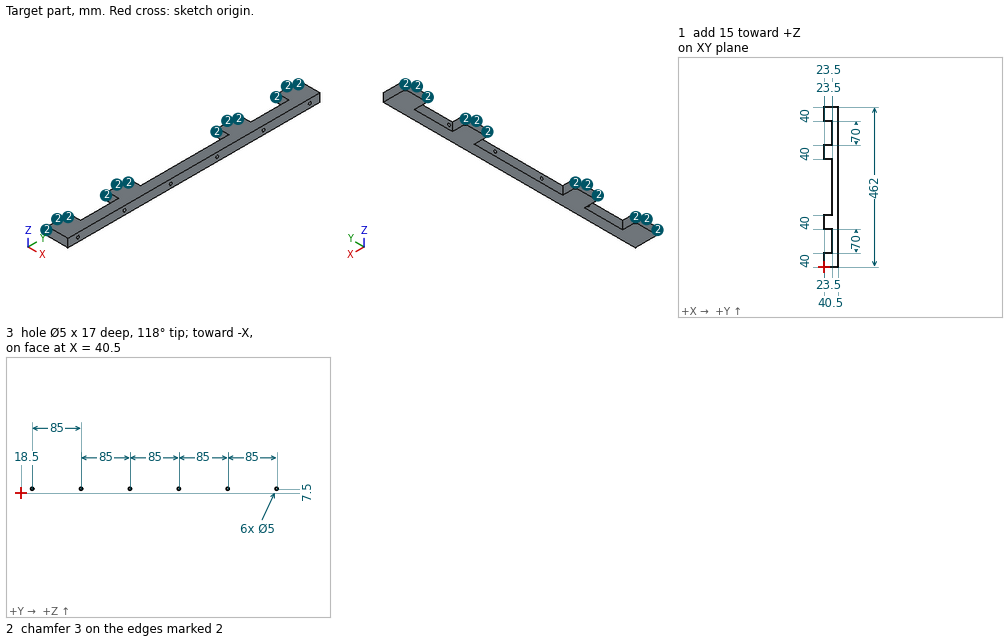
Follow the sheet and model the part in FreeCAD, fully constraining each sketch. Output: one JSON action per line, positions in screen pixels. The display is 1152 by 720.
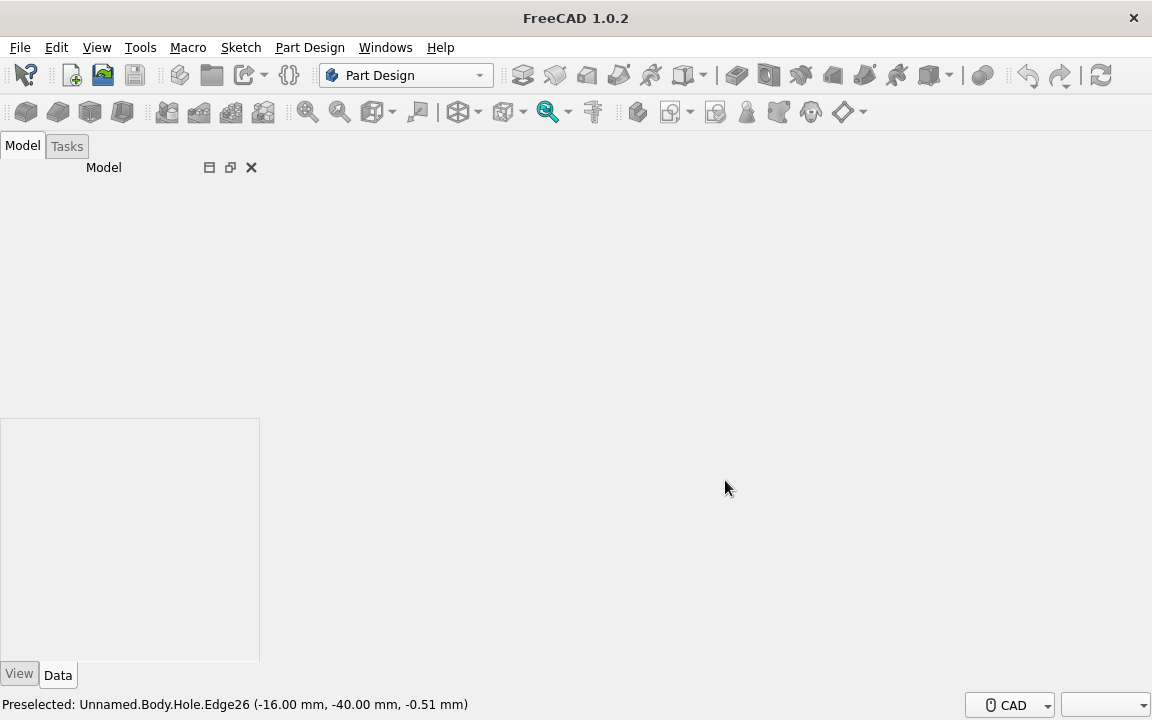
{"action": "left_click", "coordinate": [72, 76]}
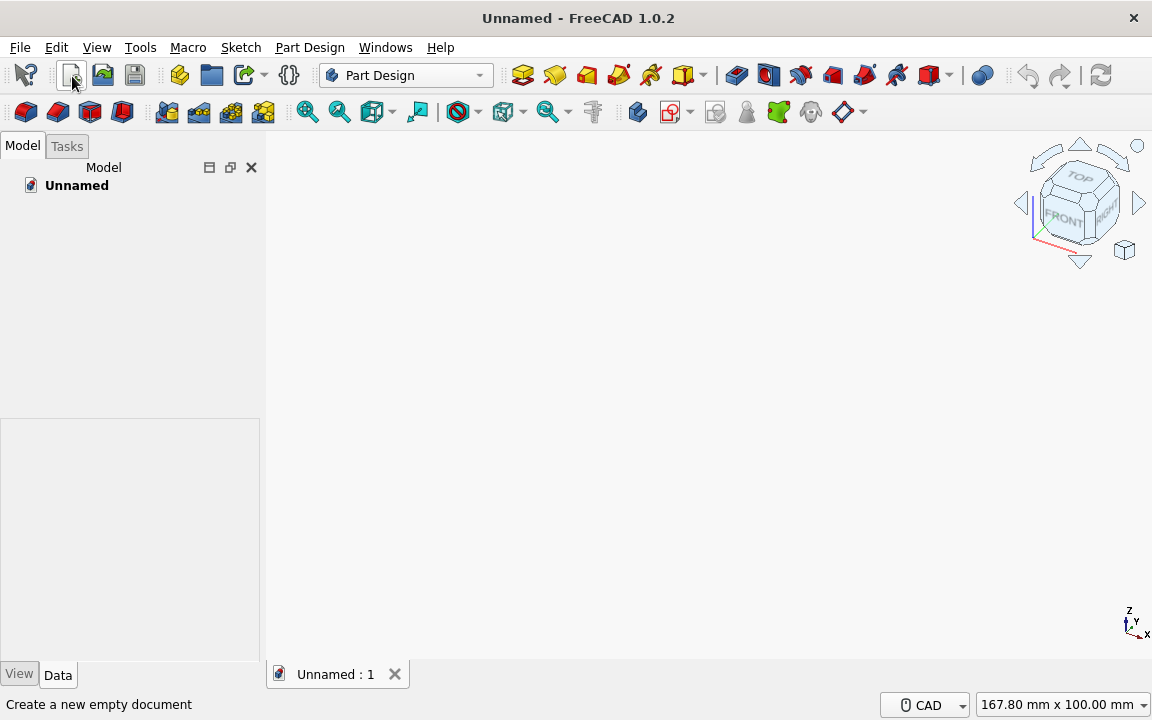
{"action": "left_click", "coordinate": [670, 112]}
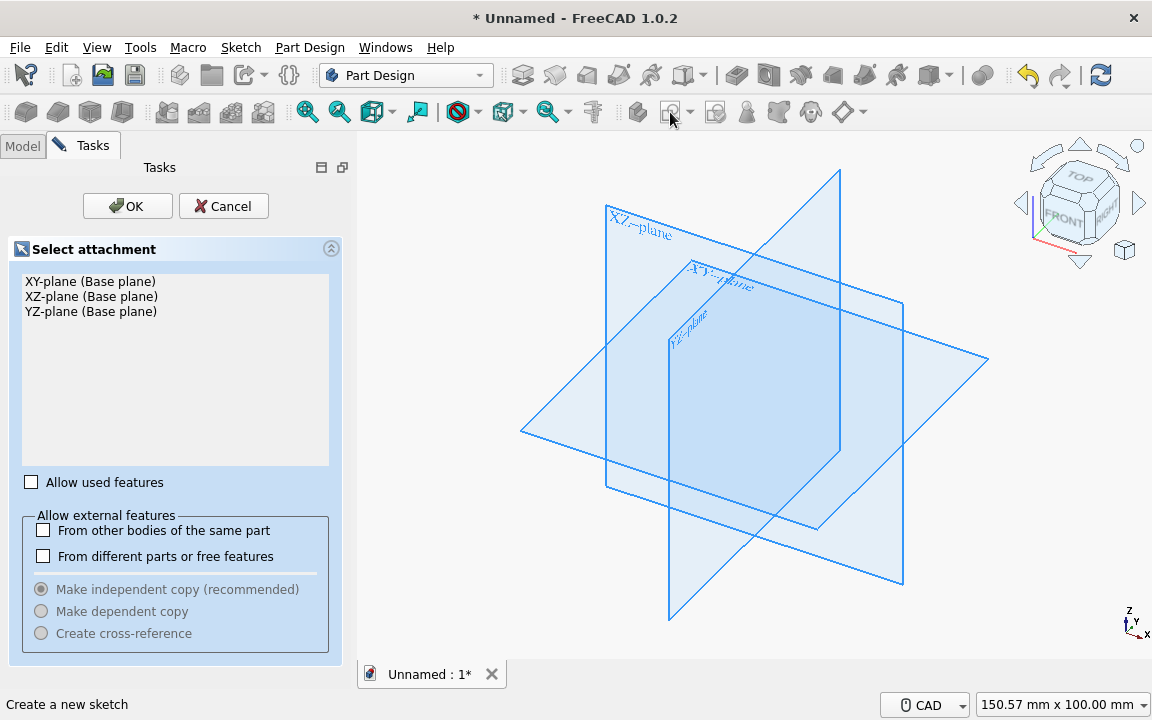
{"action": "left_click", "coordinate": [82, 282]}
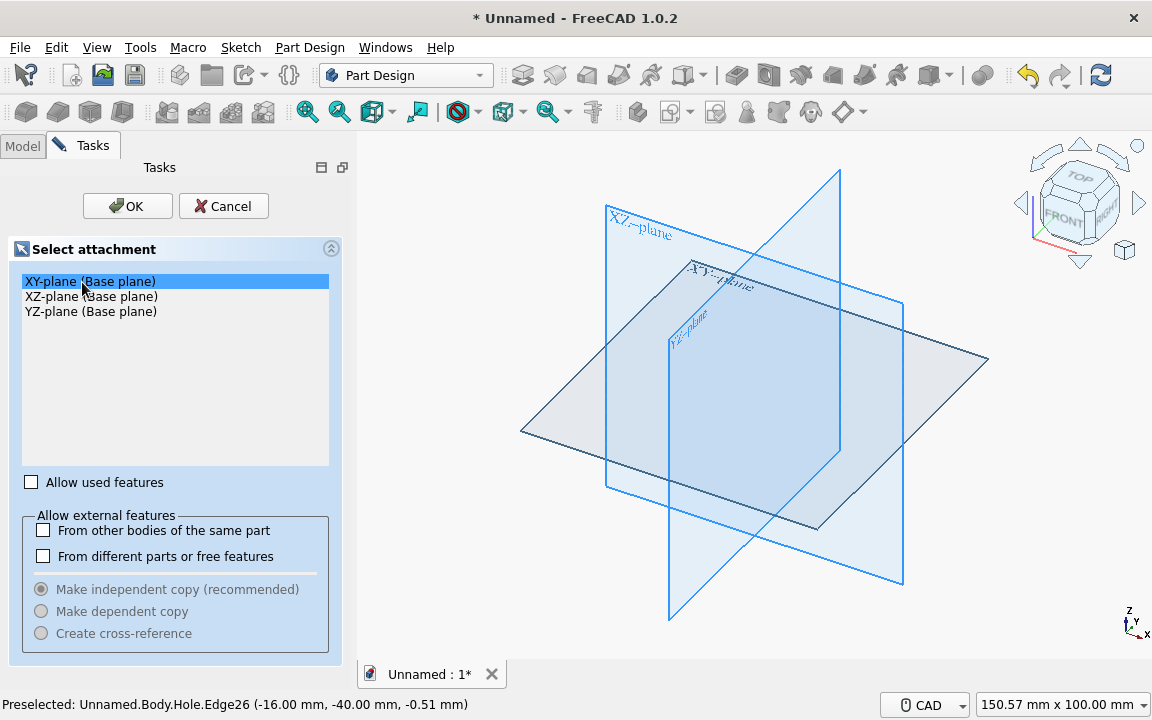
{"action": "left_click", "coordinate": [128, 206]}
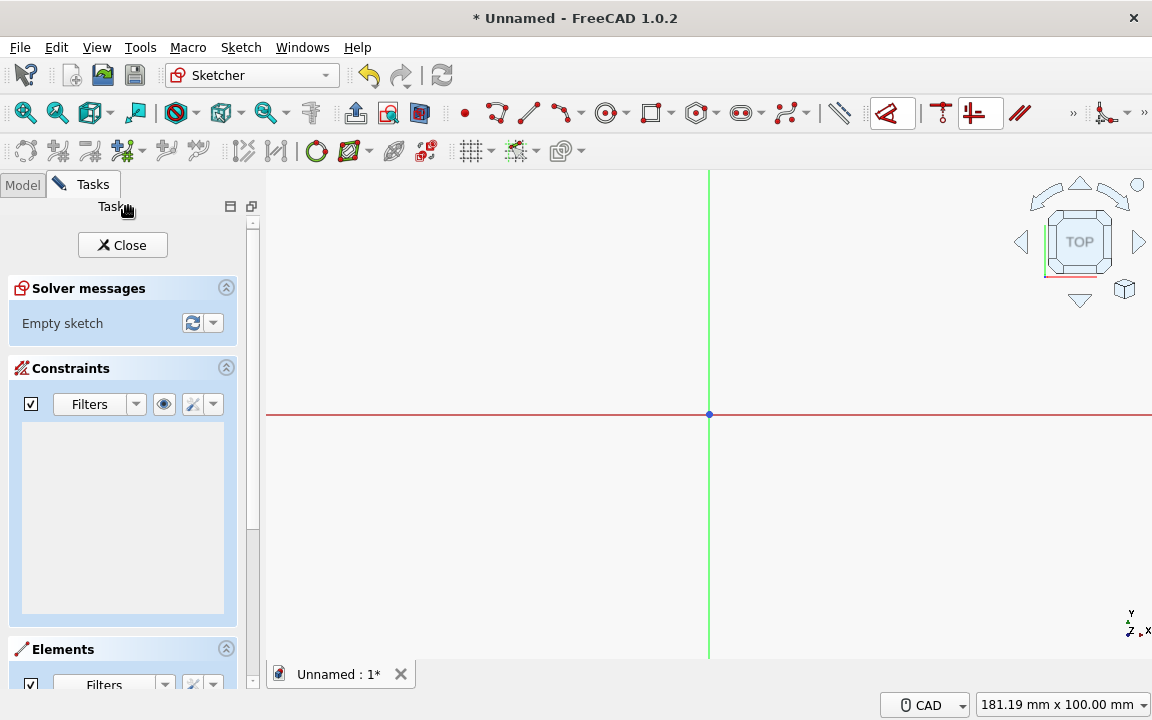
{"action": "scroll", "coordinate": [614, 591], "scroll_direction": "down", "scroll_amount": 10}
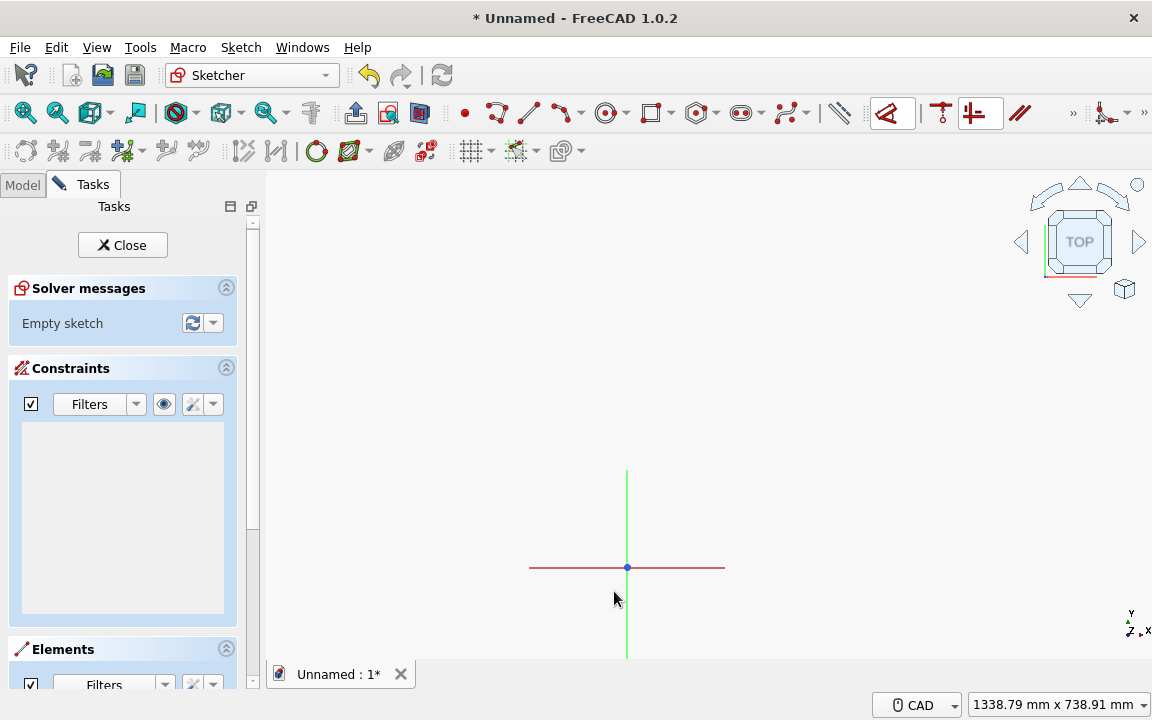
{"action": "left_click", "coordinate": [498, 114]}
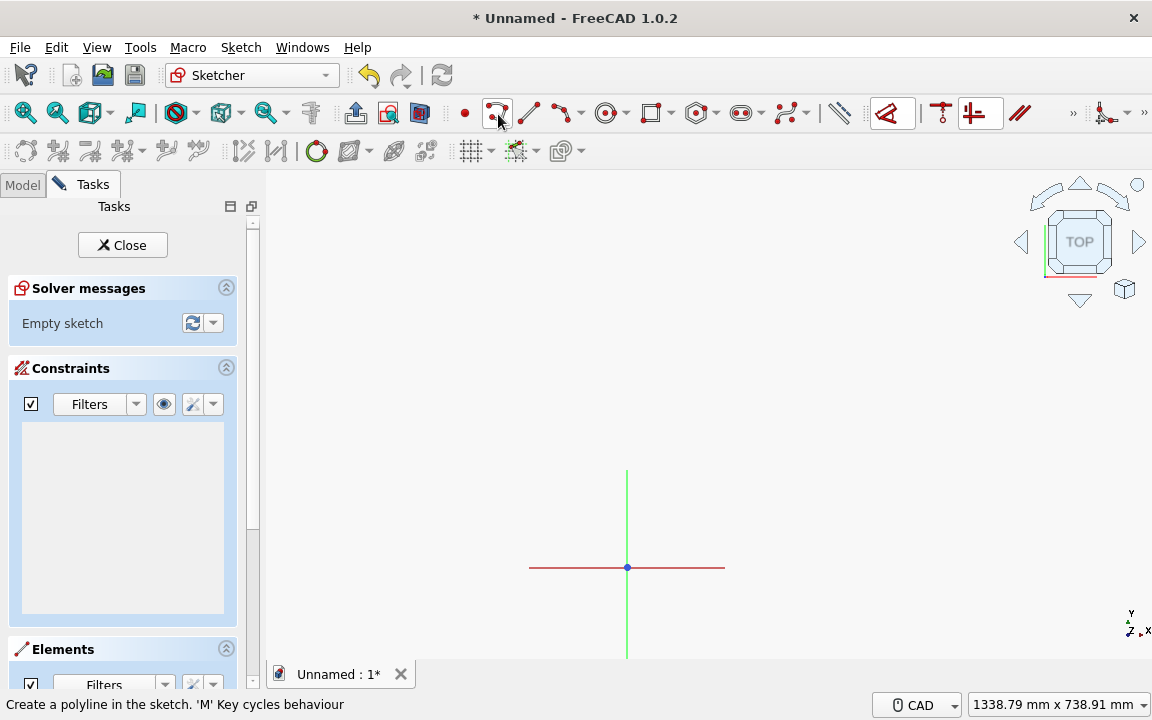
{"action": "left_click", "coordinate": [627, 568]}
{"action": "left_click", "coordinate": [654, 559]}
{"action": "left_click", "coordinate": [654, 262]}
{"action": "left_click", "coordinate": [627, 262]}
{"action": "left_click", "coordinate": [636, 289]}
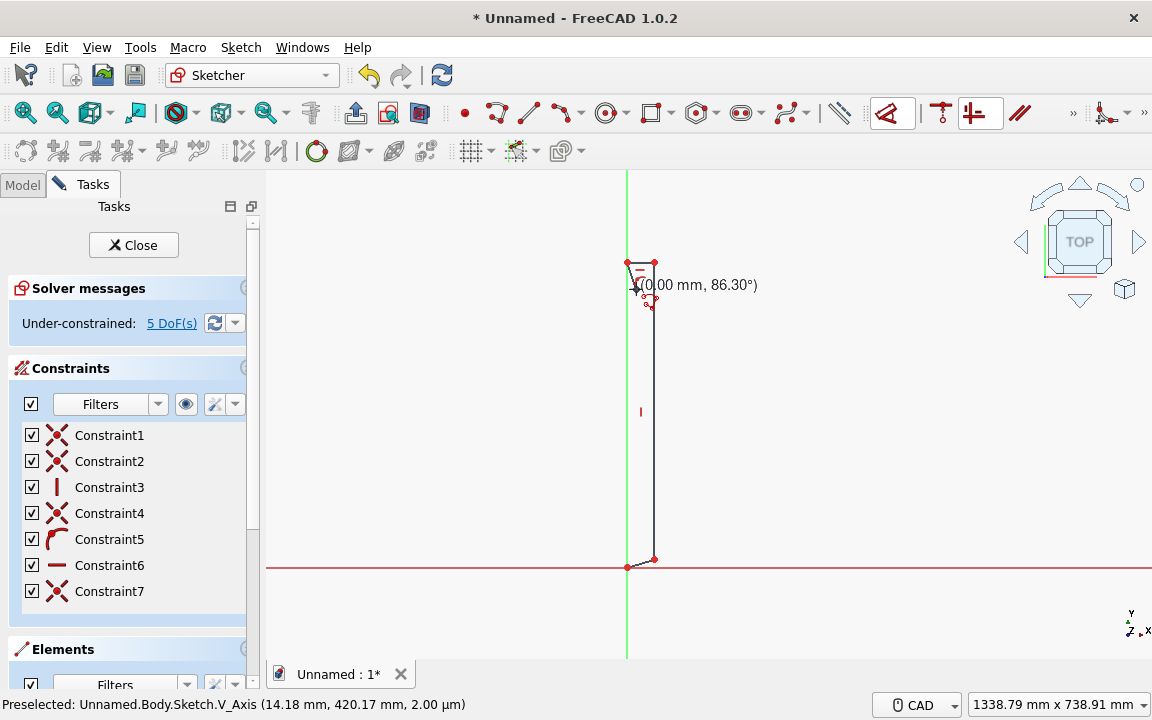
{"action": "scroll", "coordinate": [643, 289], "scroll_direction": "up", "scroll_amount": 2}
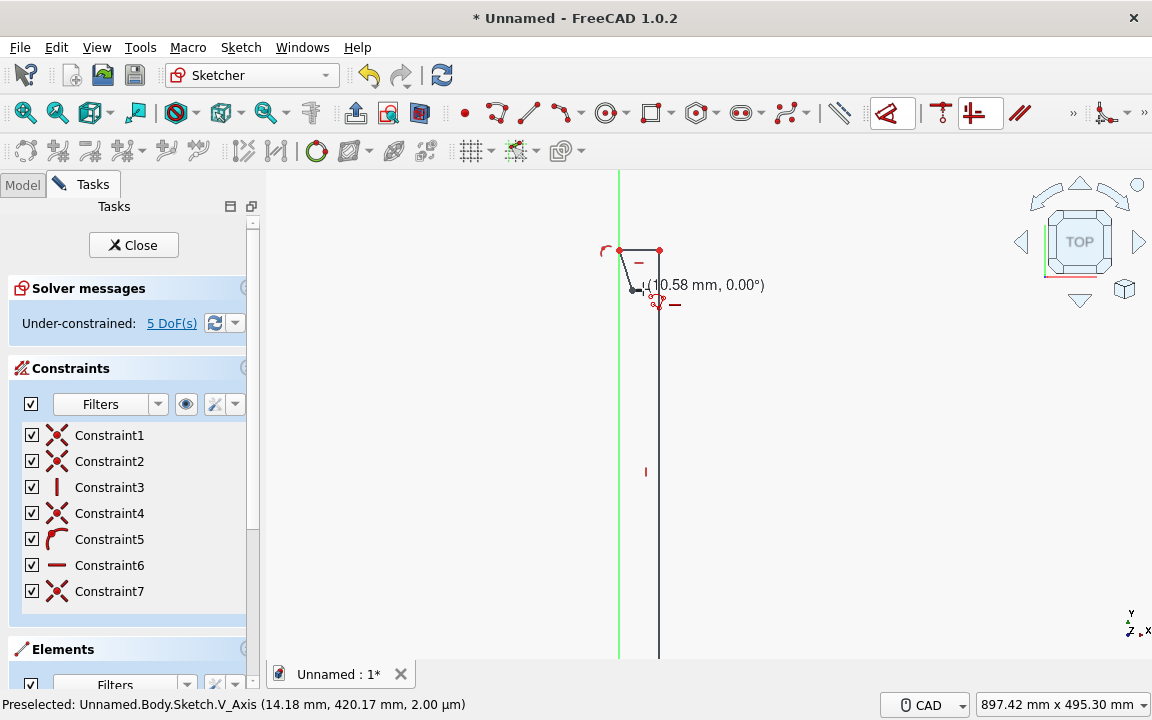
{"action": "left_click", "coordinate": [642, 289]}
{"action": "left_click", "coordinate": [642, 357]}
{"action": "left_click", "coordinate": [619, 357]}
{"action": "left_click", "coordinate": [628, 397]}
{"action": "left_click", "coordinate": [642, 397]}
{"action": "left_click", "coordinate": [642, 557]}
{"action": "left_click", "coordinate": [619, 557]}
{"action": "left_click", "coordinate": [628, 596]}
{"action": "left_click", "coordinate": [642, 596]}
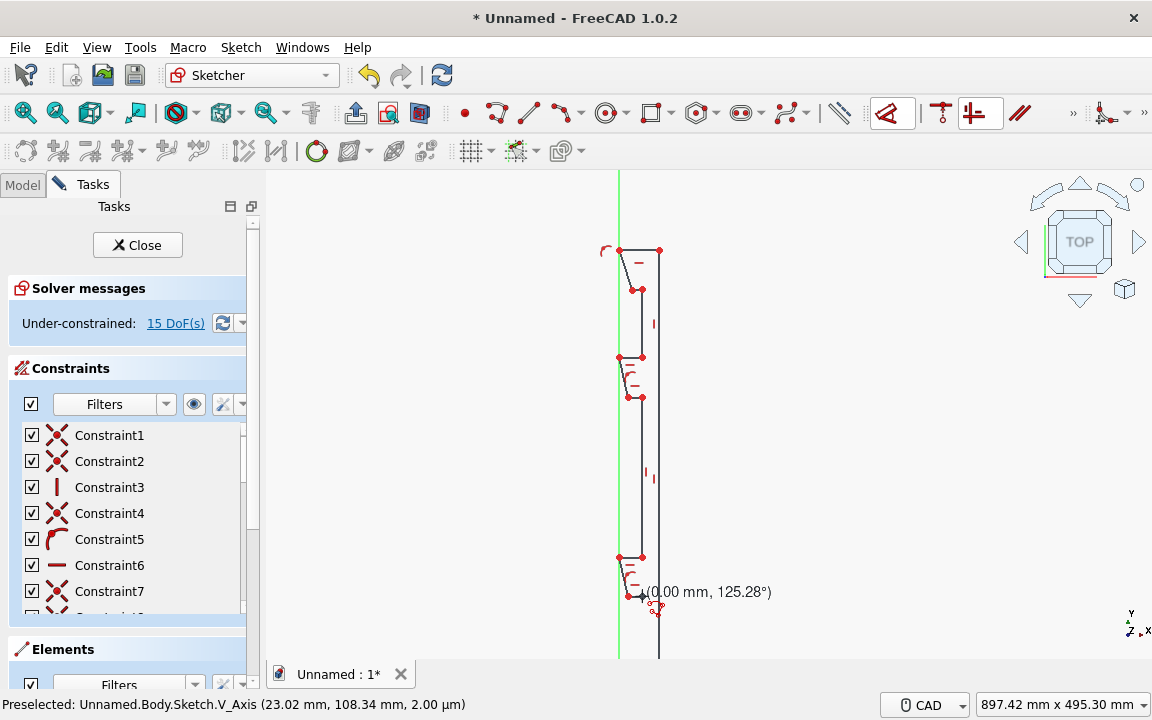
{"action": "scroll", "coordinate": [643, 288], "scroll_direction": "down", "scroll_amount": 2}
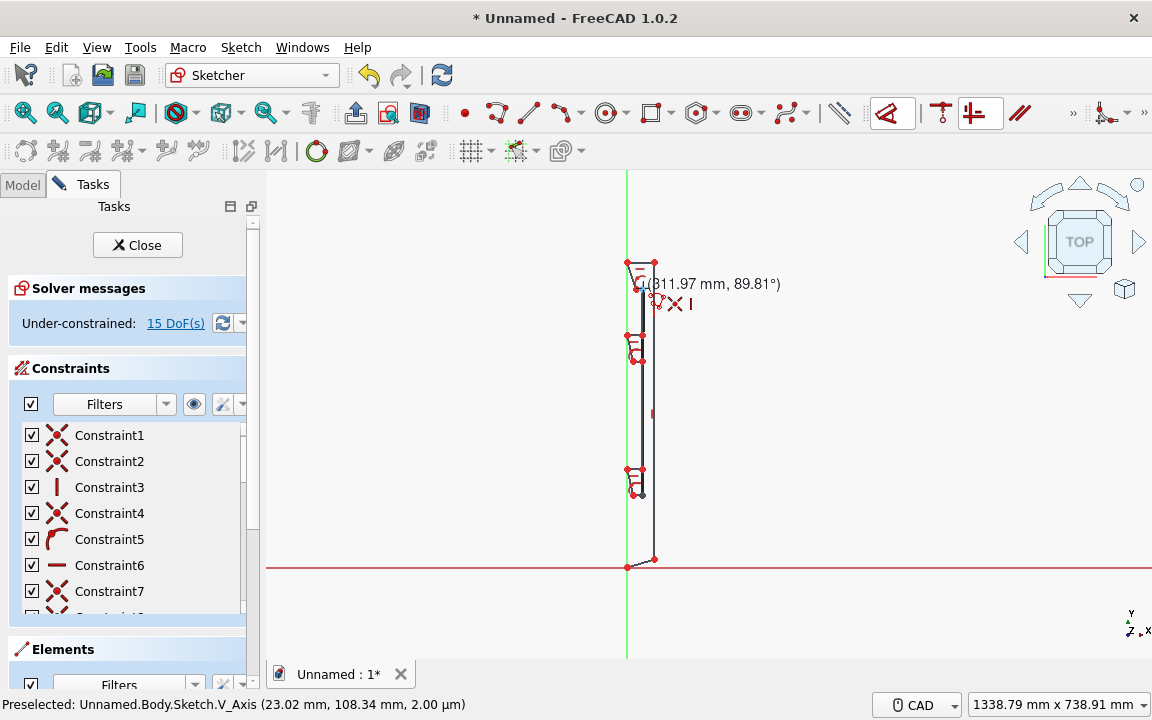
{"action": "scroll", "coordinate": [643, 541], "scroll_direction": "up", "scroll_amount": 2}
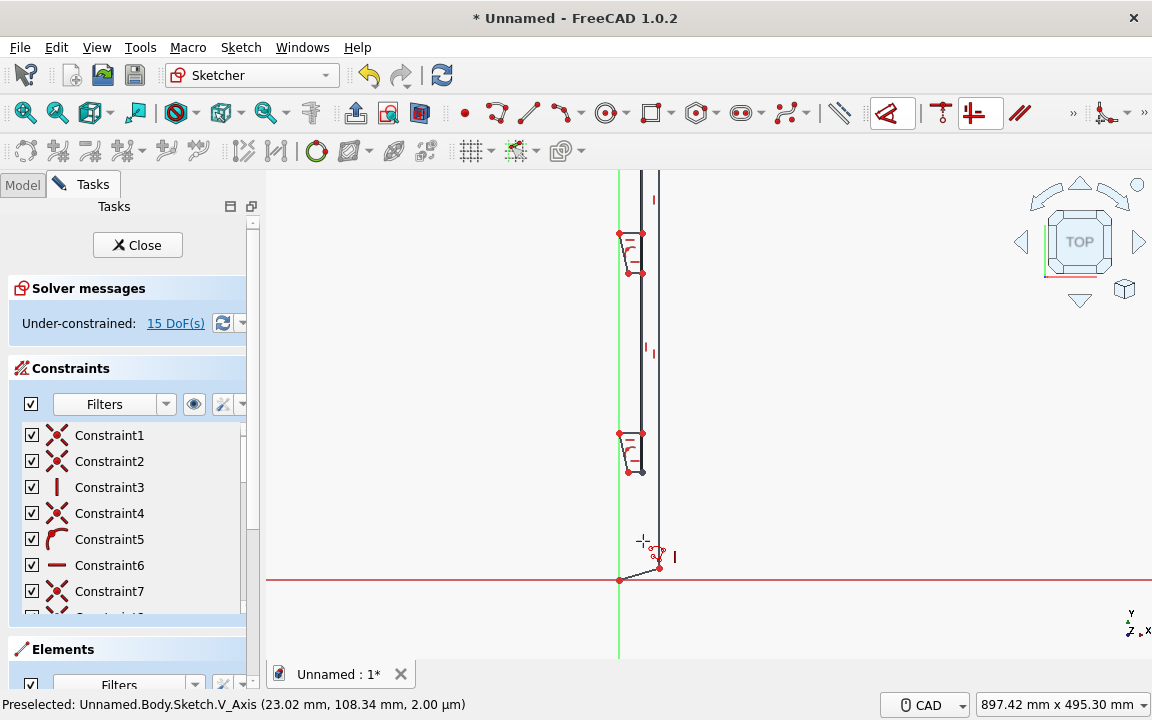
{"action": "left_click", "coordinate": [642, 541]}
{"action": "left_click", "coordinate": [628, 541]}
{"action": "left_click", "coordinate": [619, 580]}
{"action": "key", "text": "Escape"}
{"action": "key", "text": "Escape"}